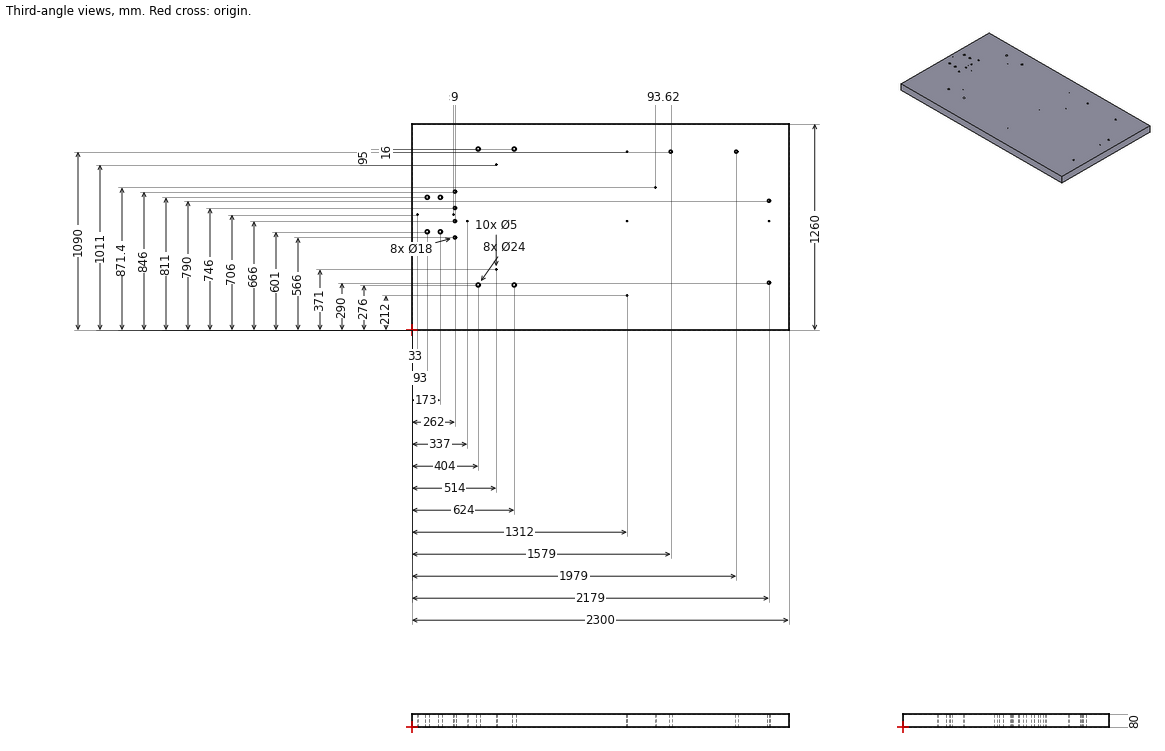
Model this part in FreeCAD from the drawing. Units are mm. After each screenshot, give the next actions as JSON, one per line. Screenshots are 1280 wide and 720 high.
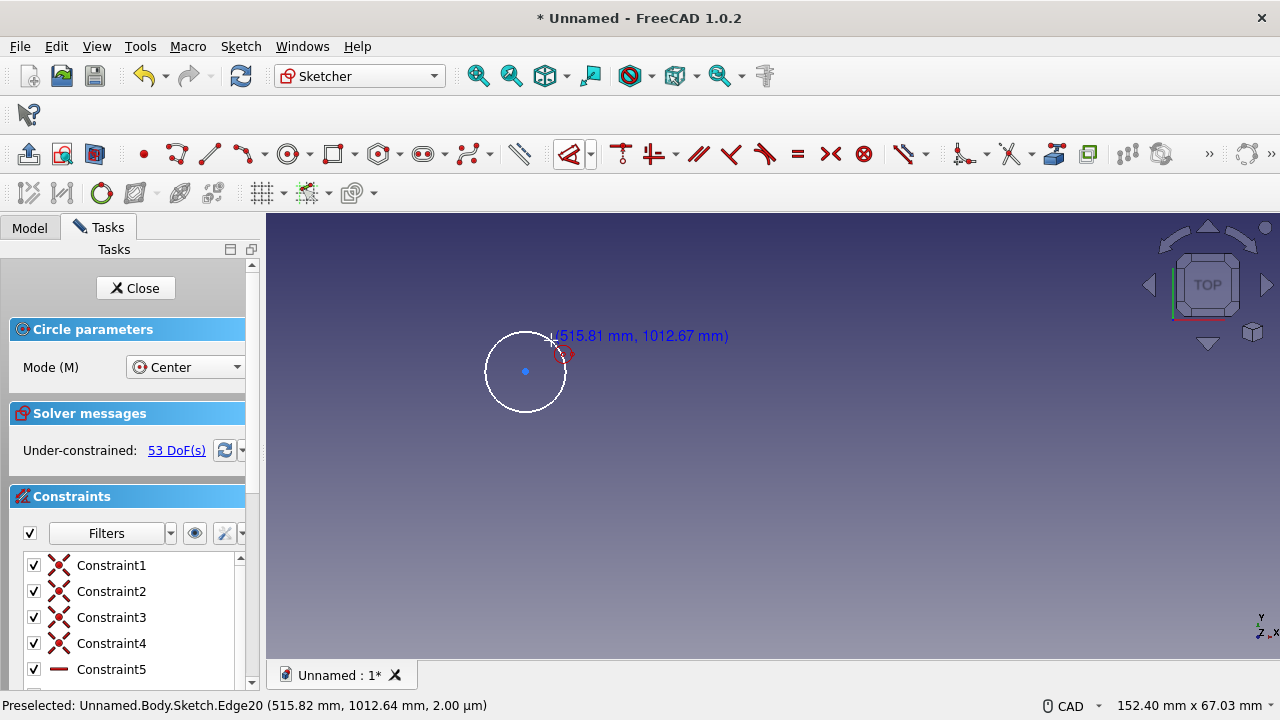
{"action": "scroll", "coordinate": [564, 351], "scroll_direction": "down", "scroll_amount": 17}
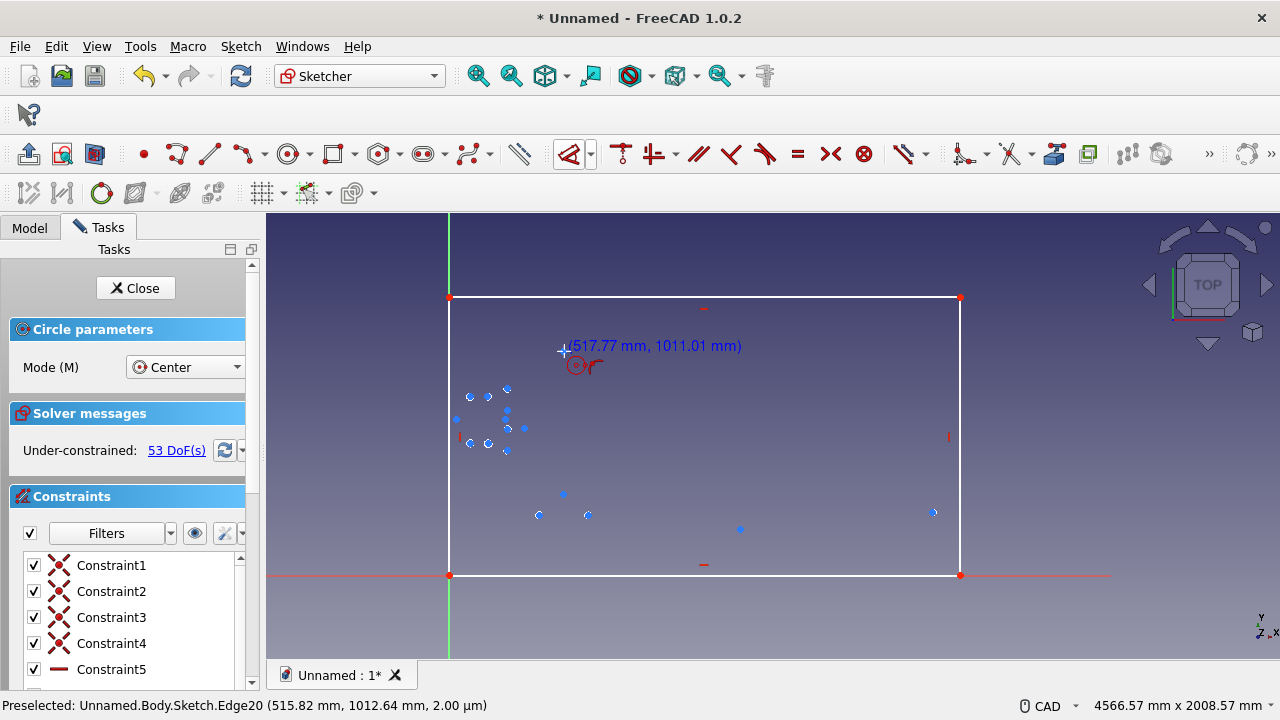
{"action": "scroll", "coordinate": [539, 330], "scroll_direction": "up", "scroll_amount": 11}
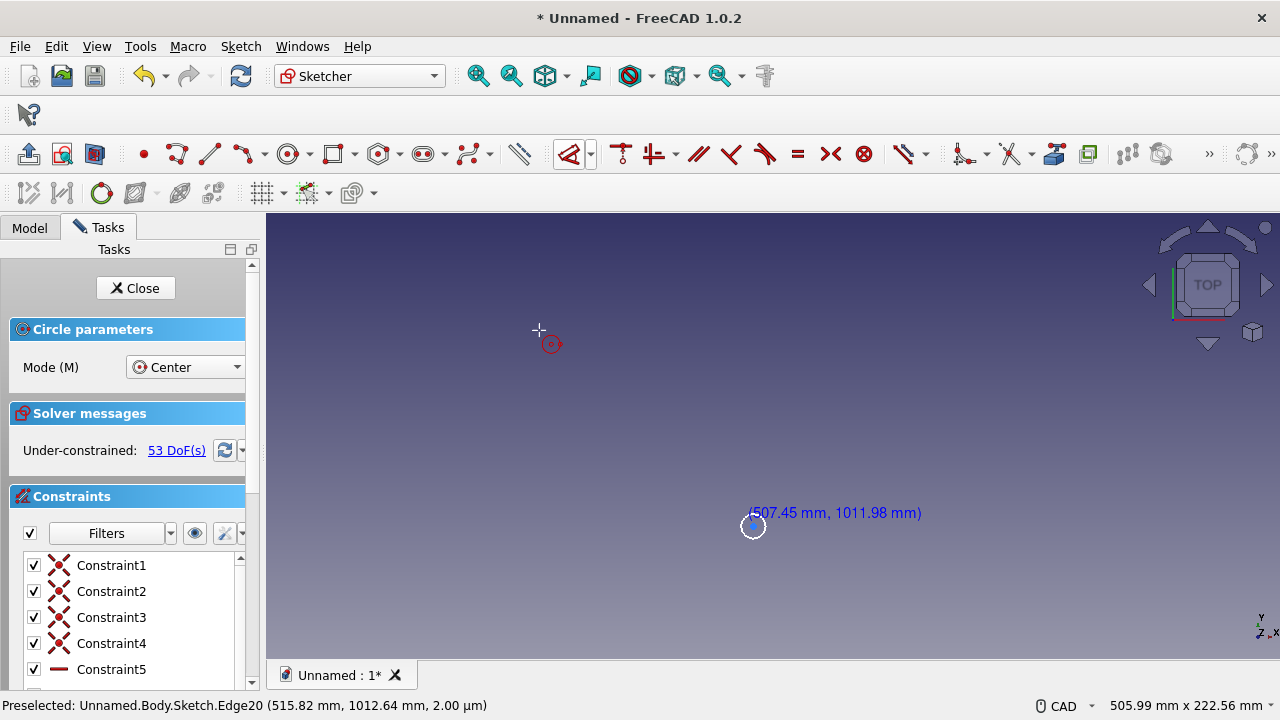
{"action": "scroll", "coordinate": [539, 330], "scroll_direction": "down", "scroll_amount": 11}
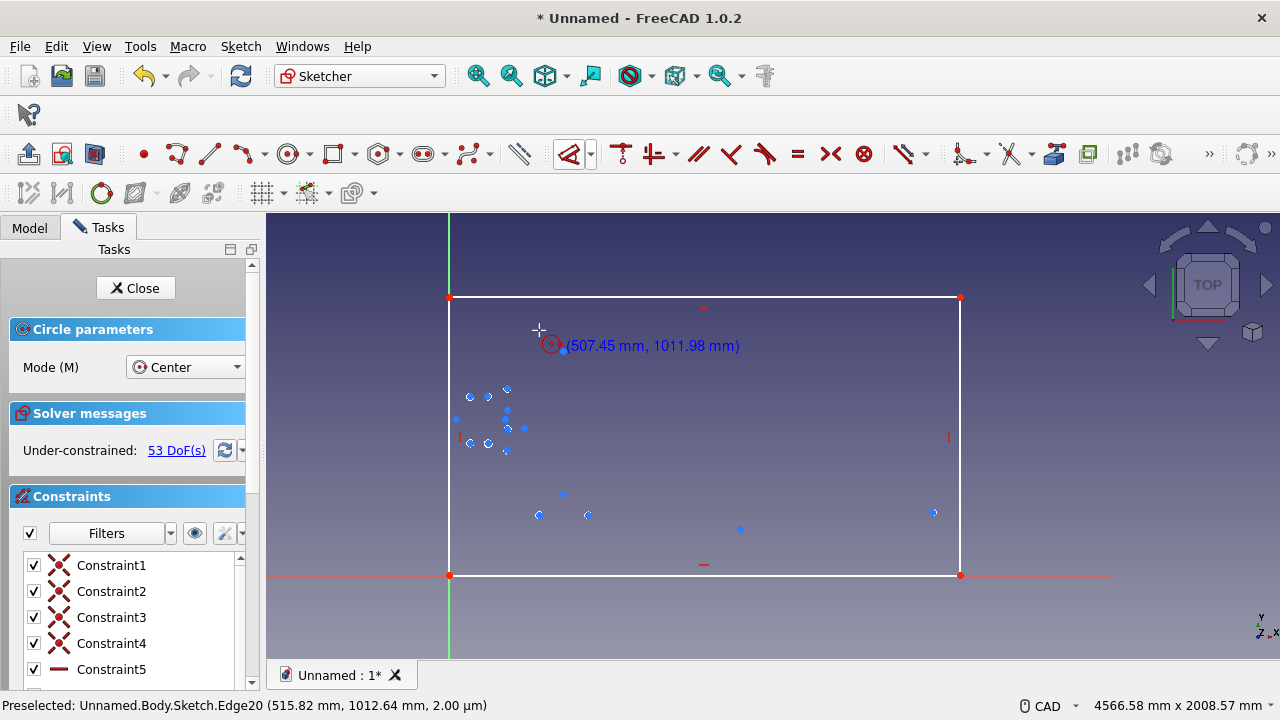
{"action": "left_click", "coordinate": [539, 330]}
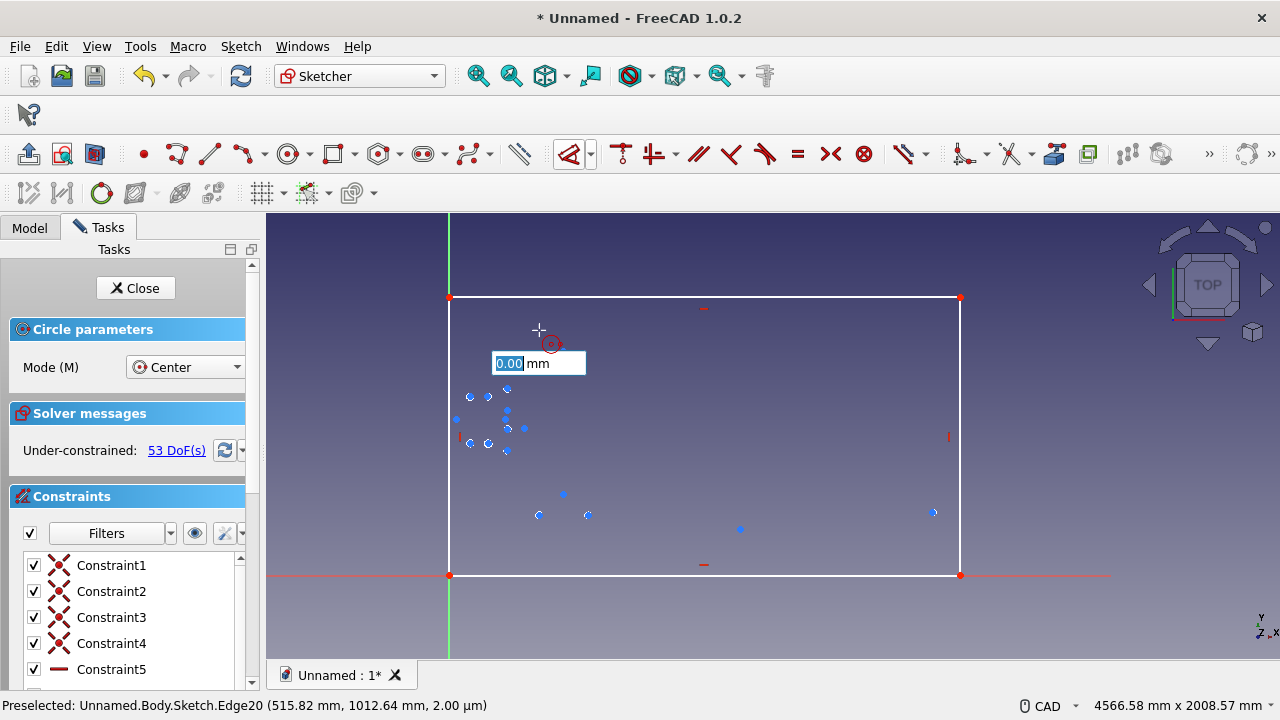
{"action": "scroll", "coordinate": [541, 328], "scroll_direction": "up", "scroll_amount": 9}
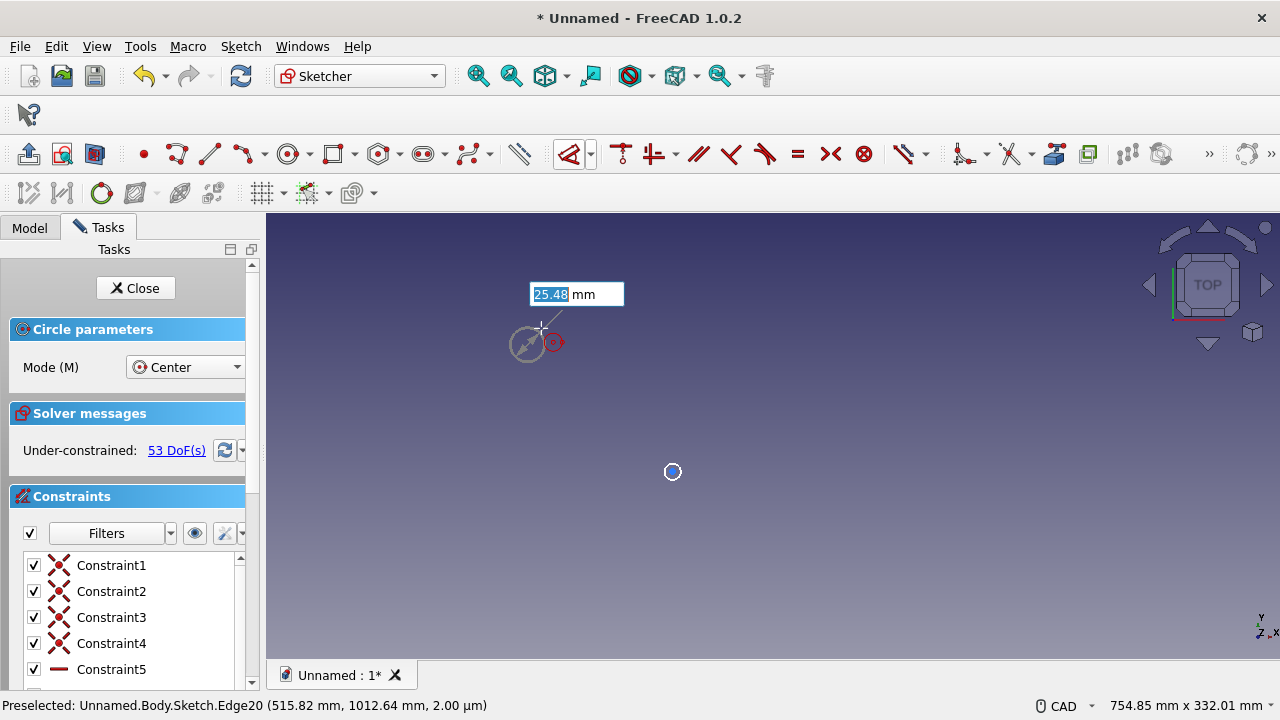
{"action": "left_click", "coordinate": [539, 329]}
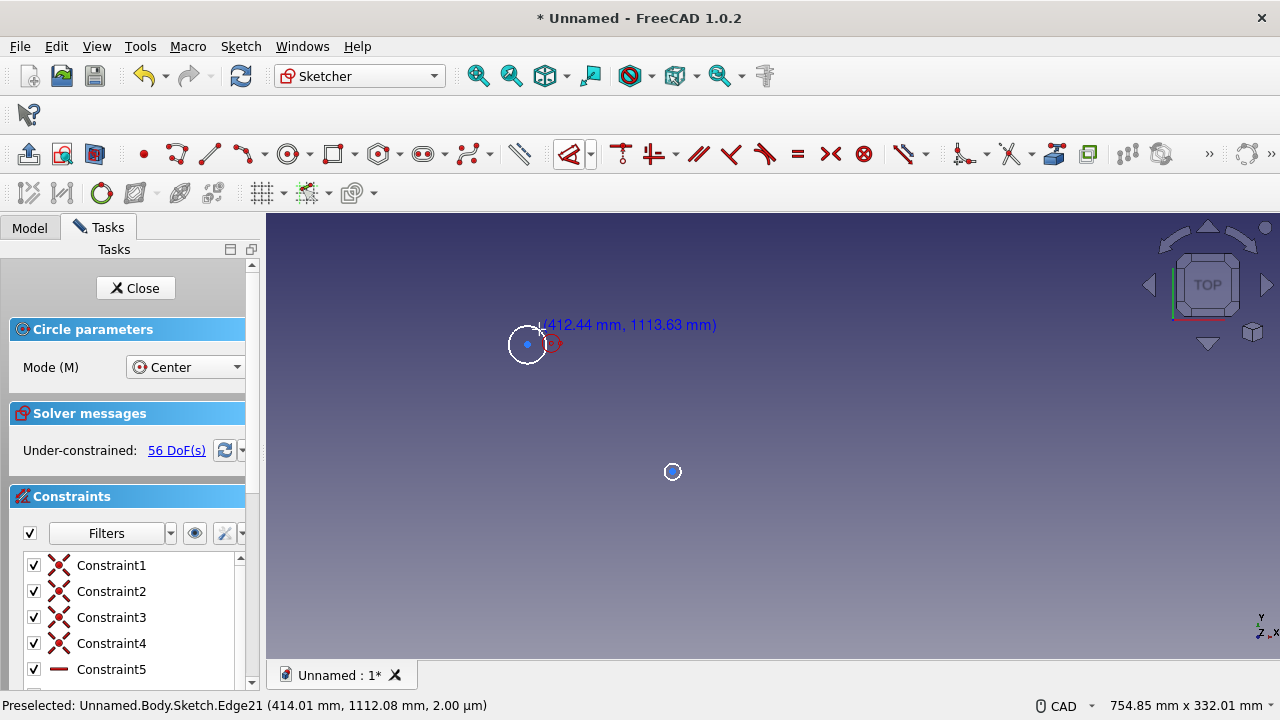
{"action": "scroll", "coordinate": [823, 340], "scroll_direction": "up", "scroll_amount": 2}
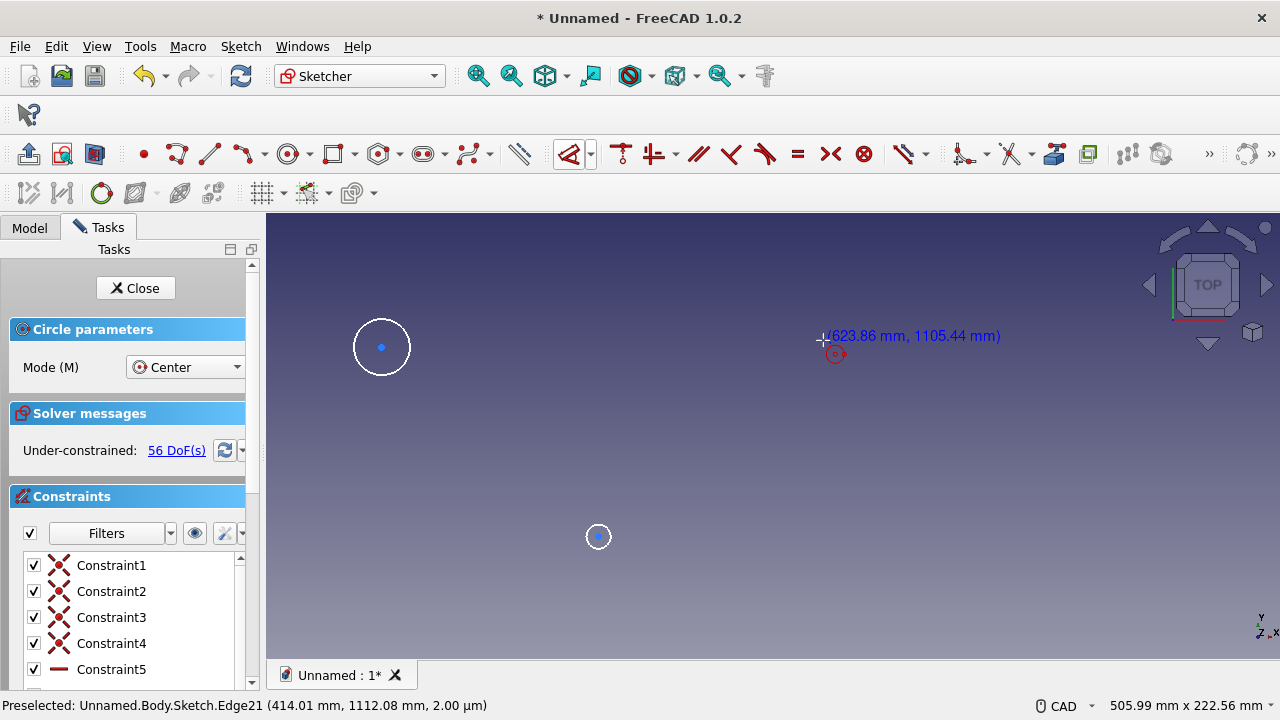
{"action": "scroll", "coordinate": [558, 329], "scroll_direction": "down", "scroll_amount": 11}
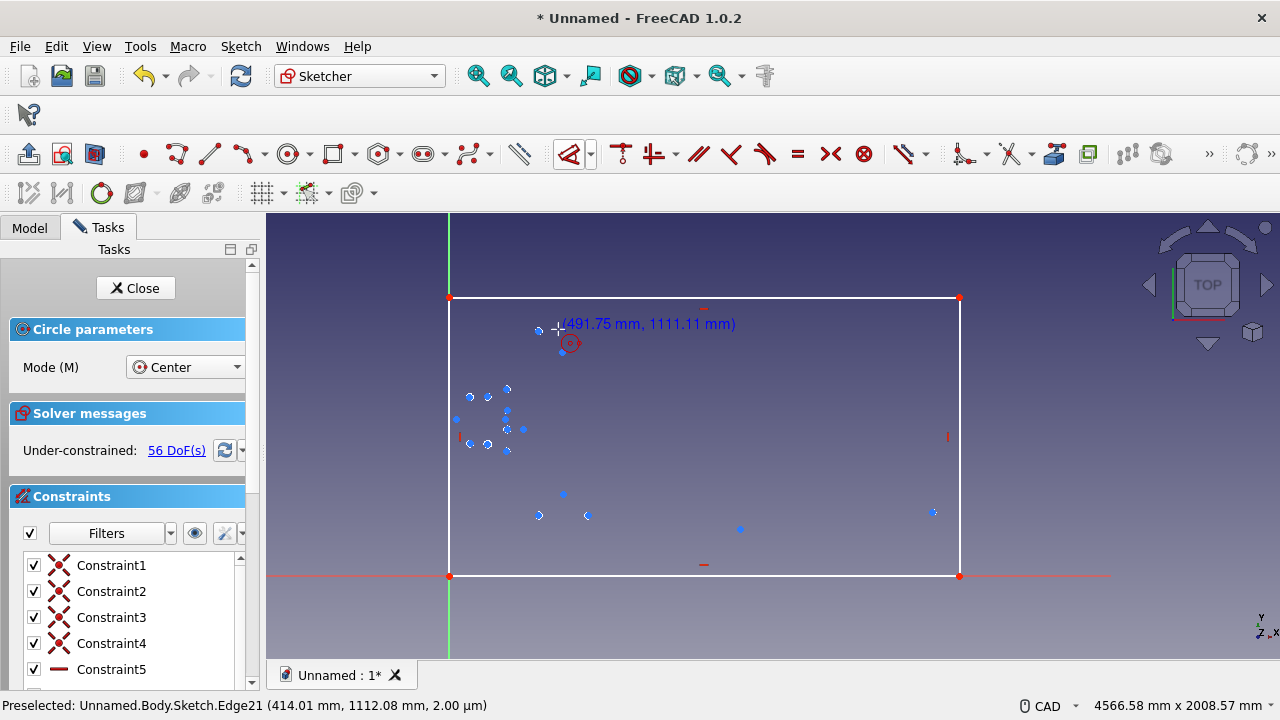
{"action": "left_click", "coordinate": [588, 330]}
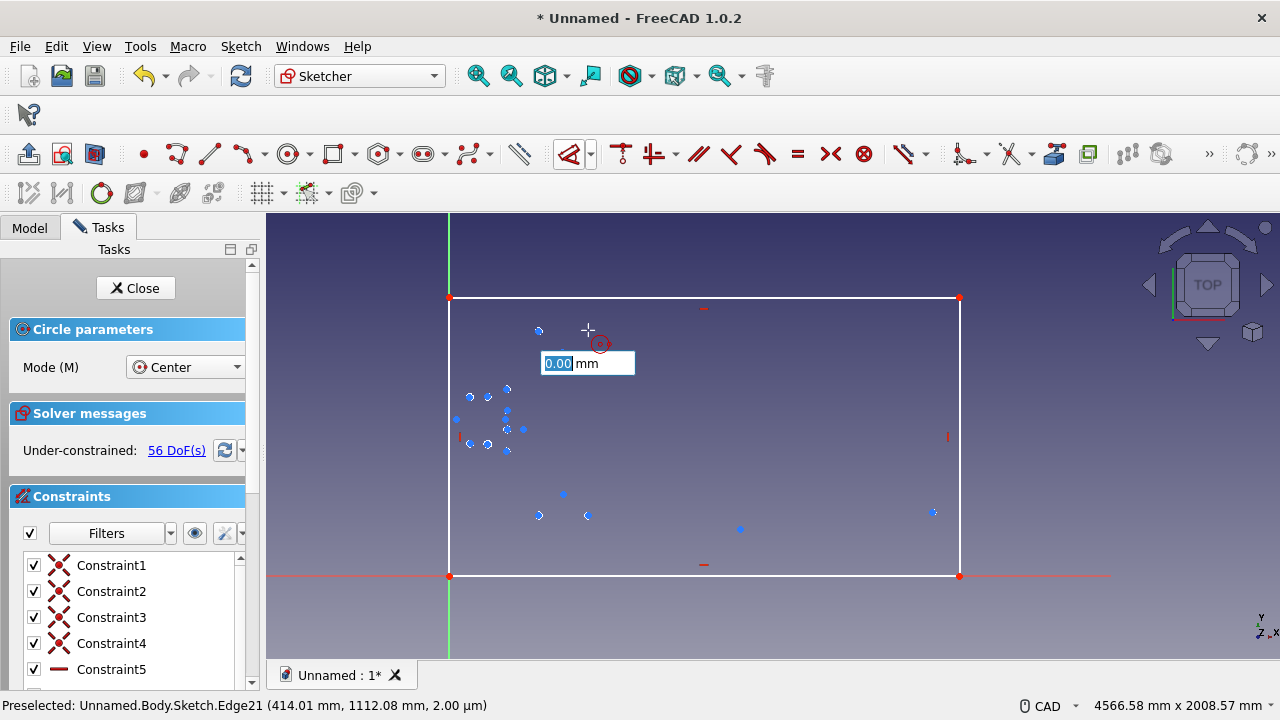
{"action": "scroll", "coordinate": [590, 329], "scroll_direction": "up", "scroll_amount": 9}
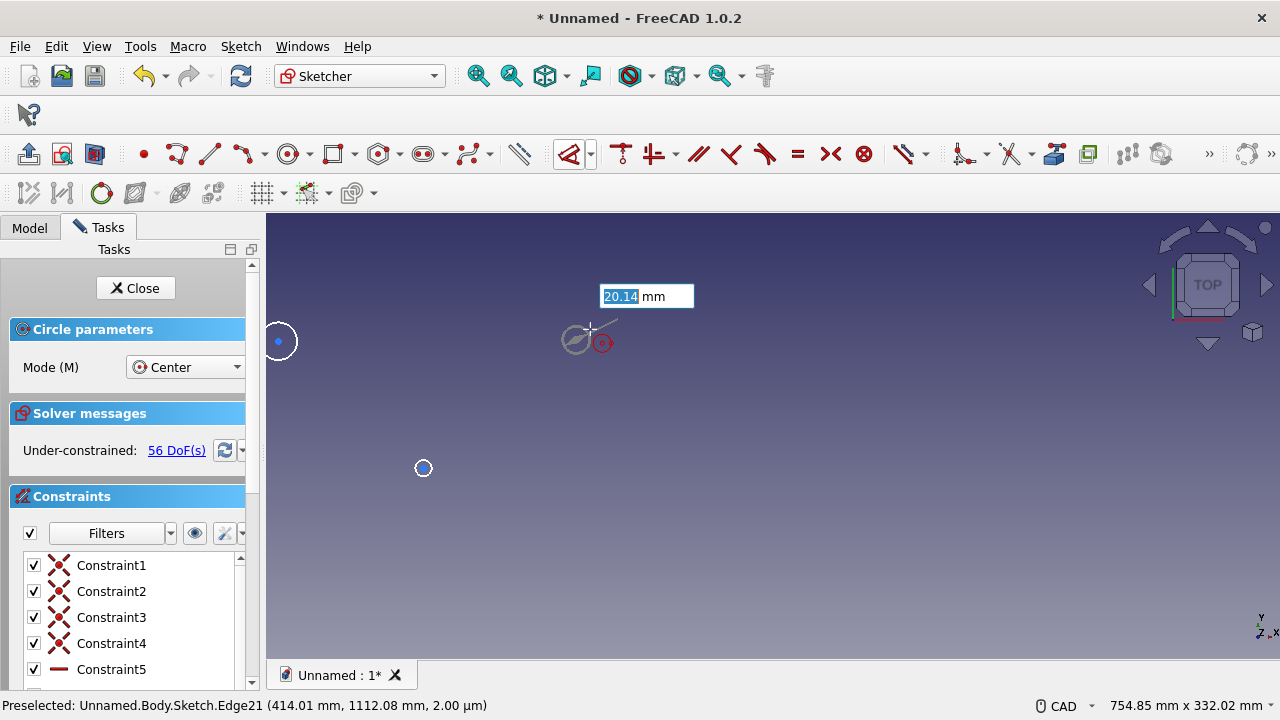
{"action": "left_click", "coordinate": [585, 325]}